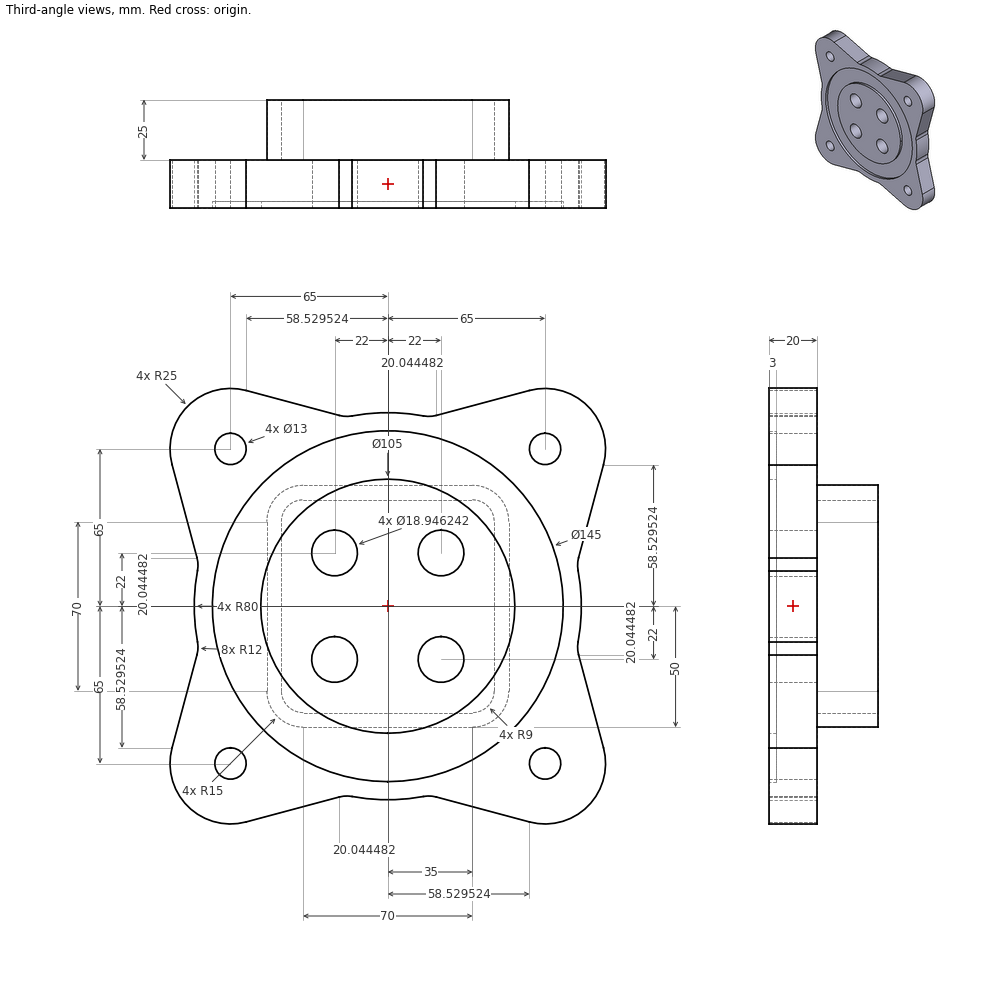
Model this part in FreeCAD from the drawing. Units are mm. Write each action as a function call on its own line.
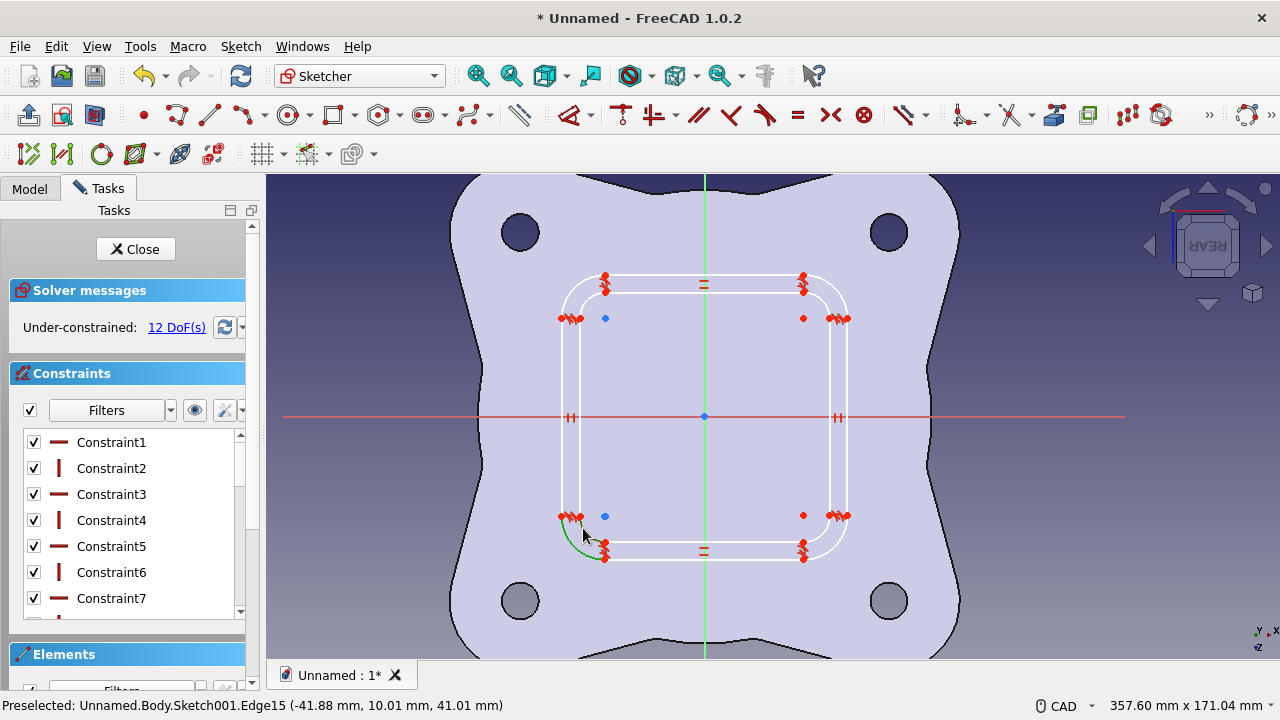
click(621, 116)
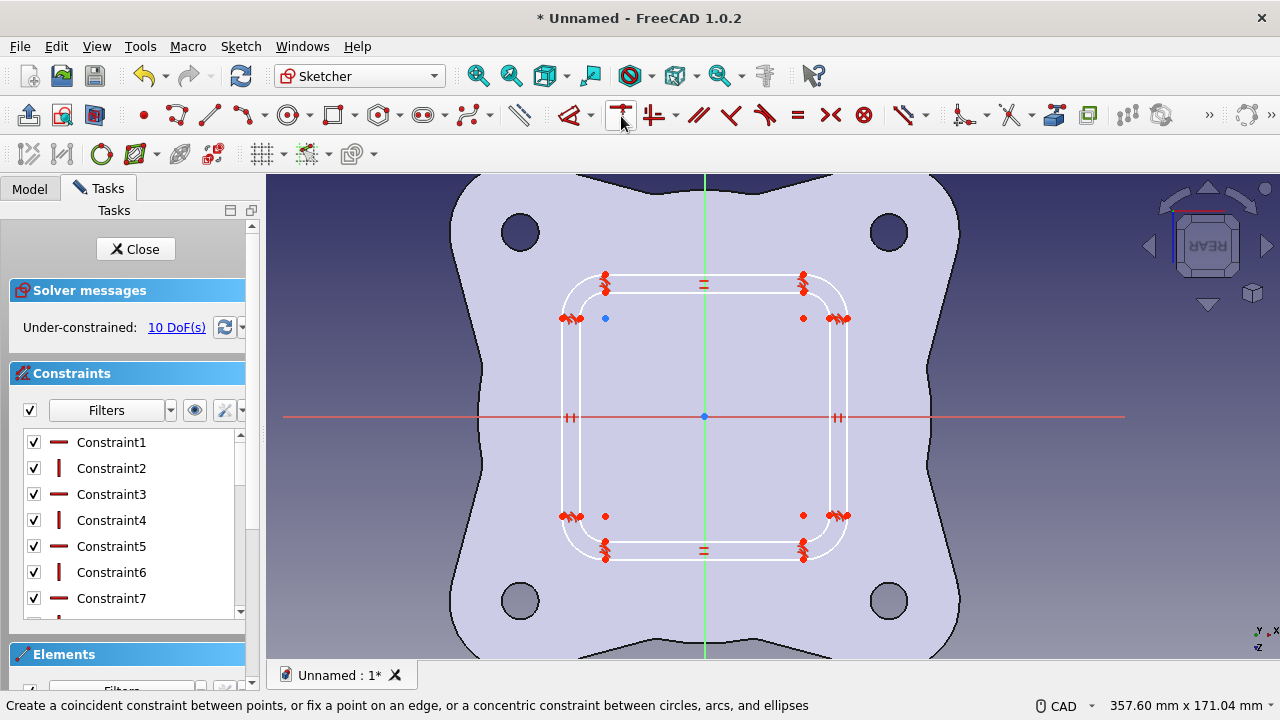
click(586, 280)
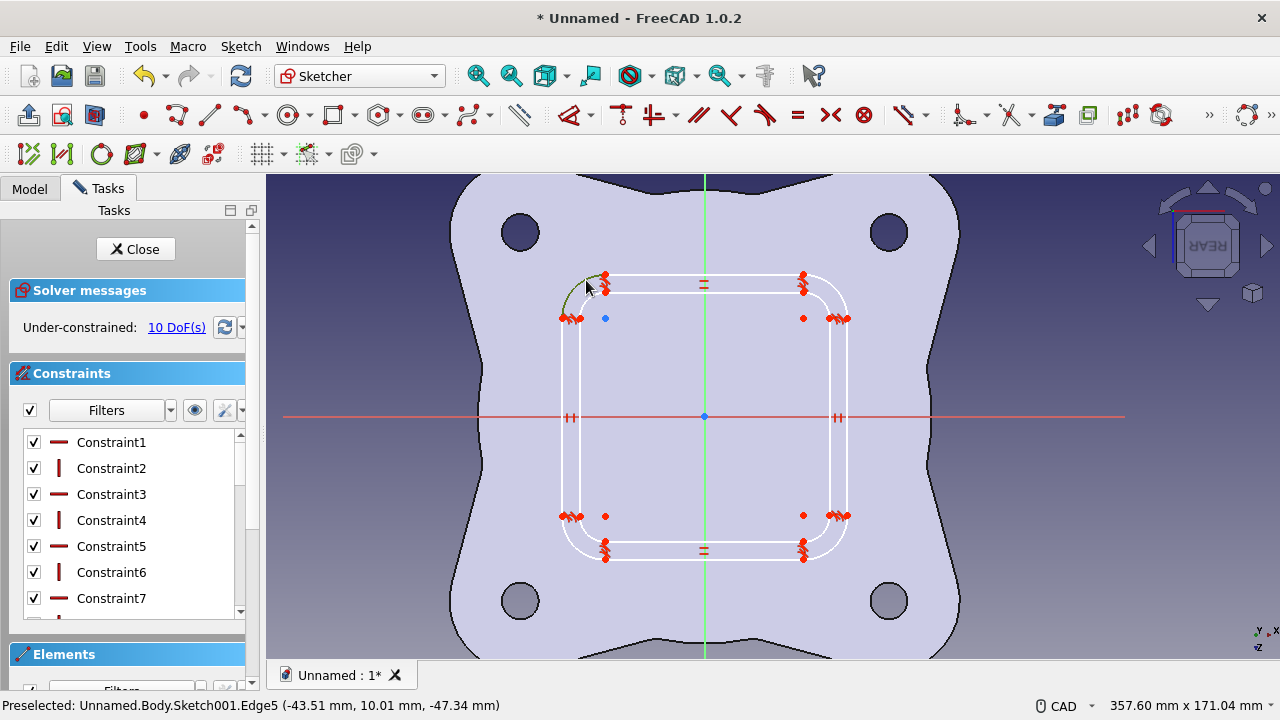
click(567, 536)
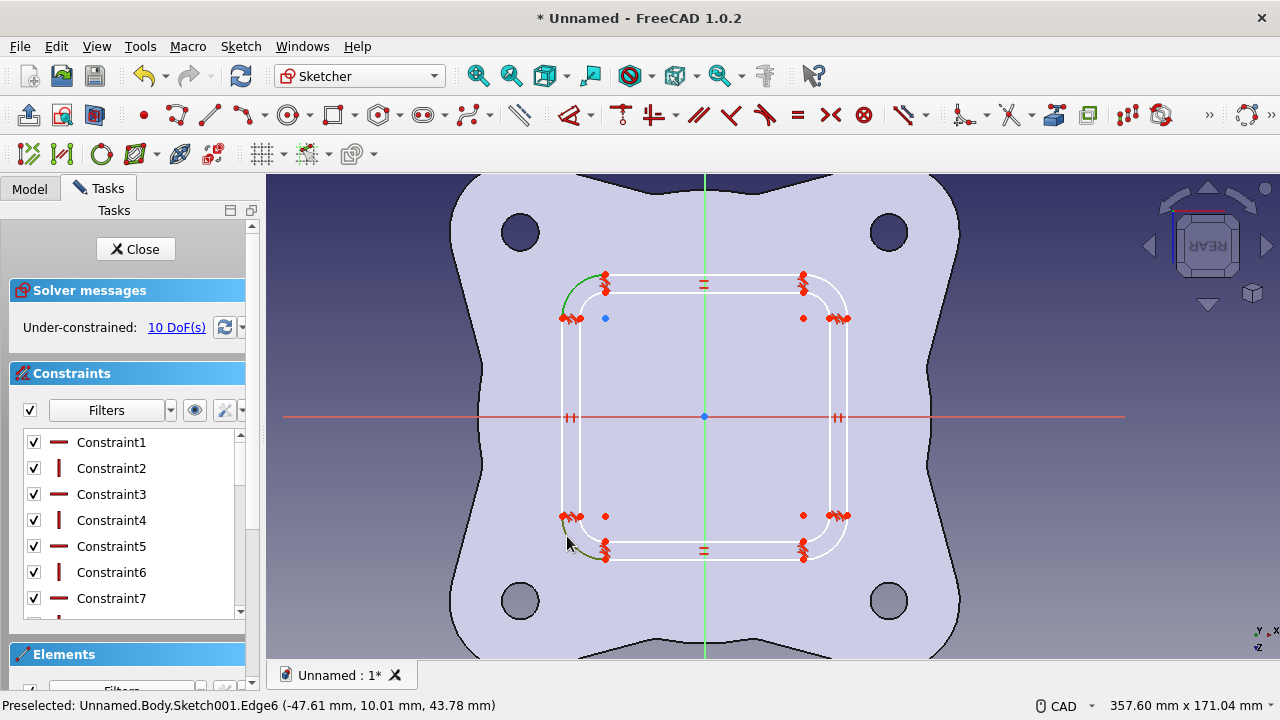
click(824, 555)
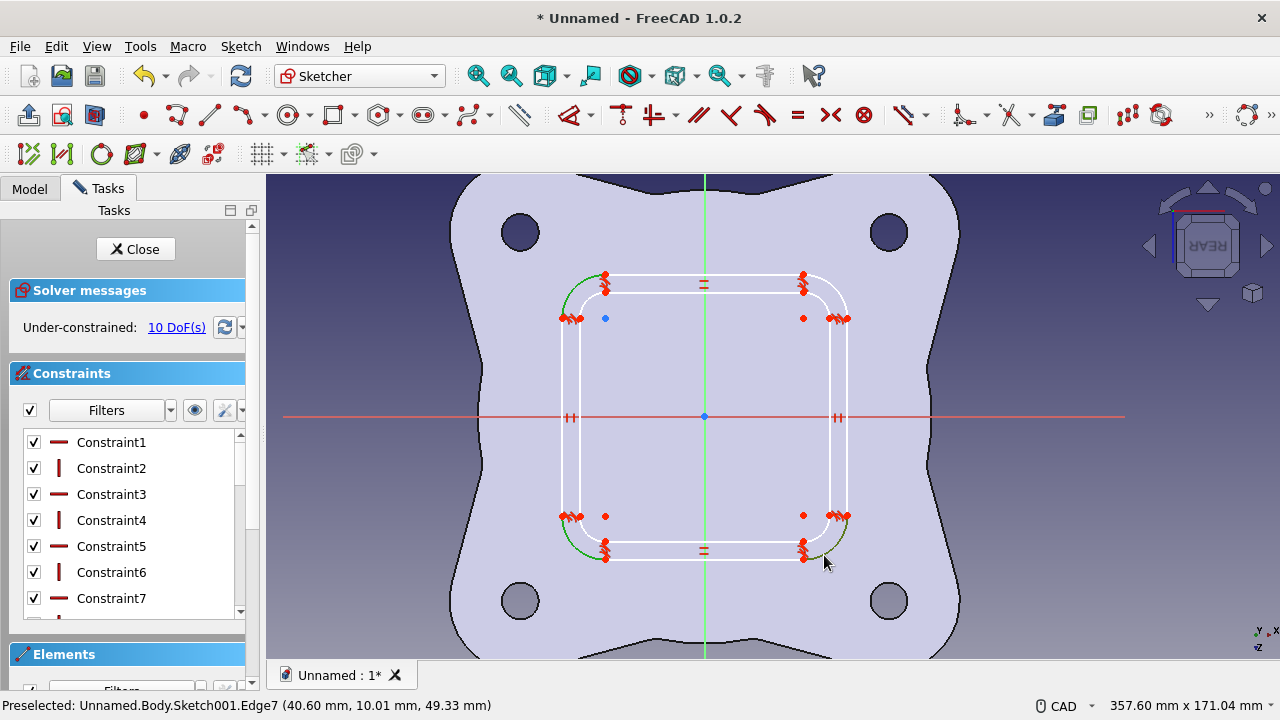
click(843, 299)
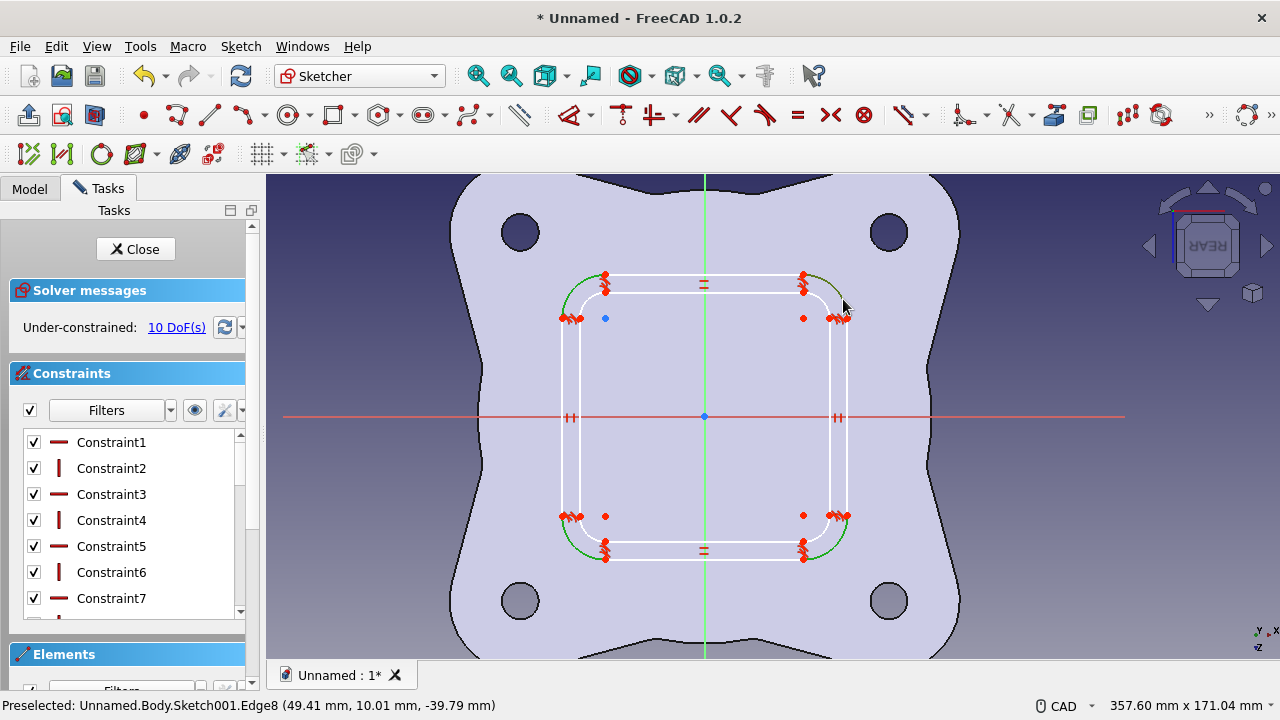
click(798, 116)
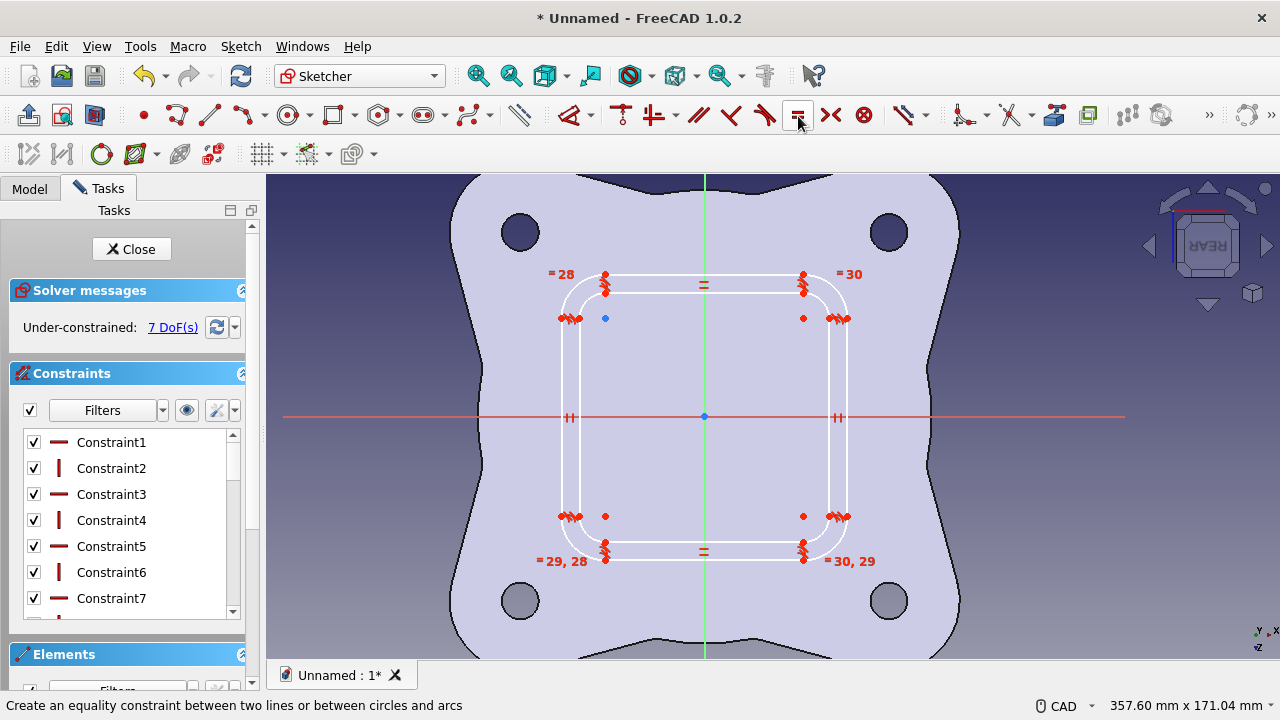
click(826, 307)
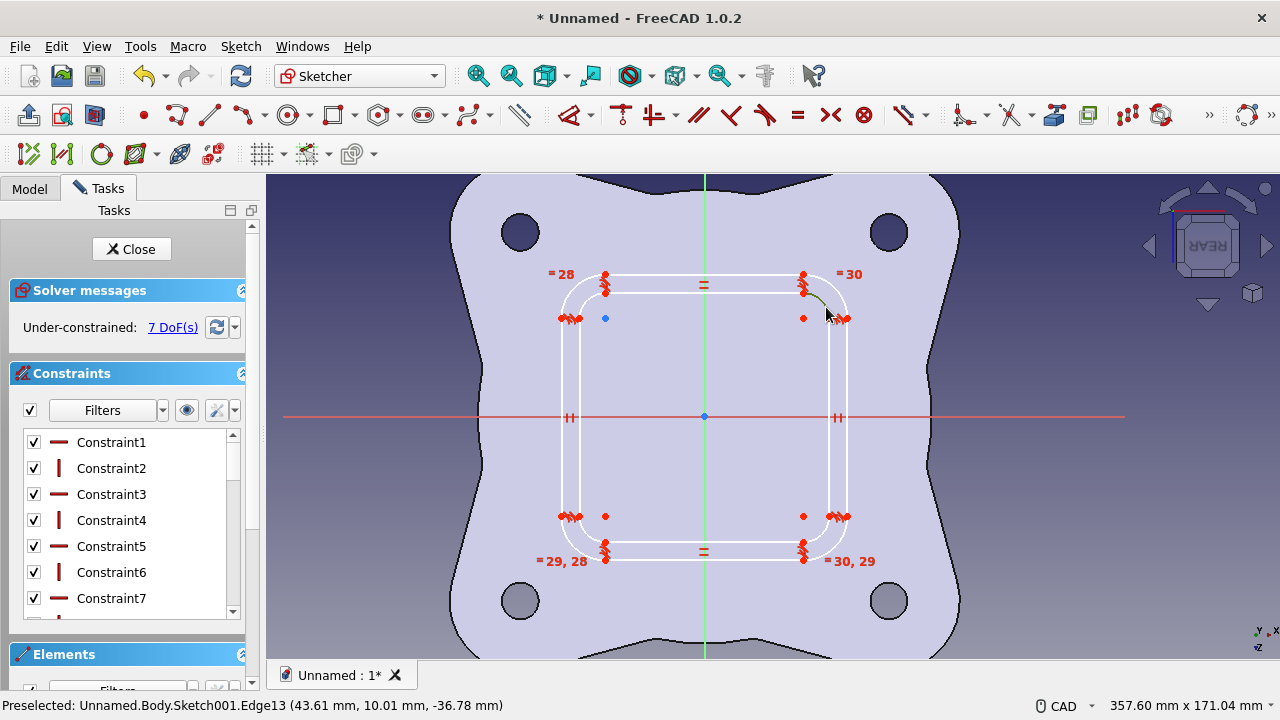
click(594, 296)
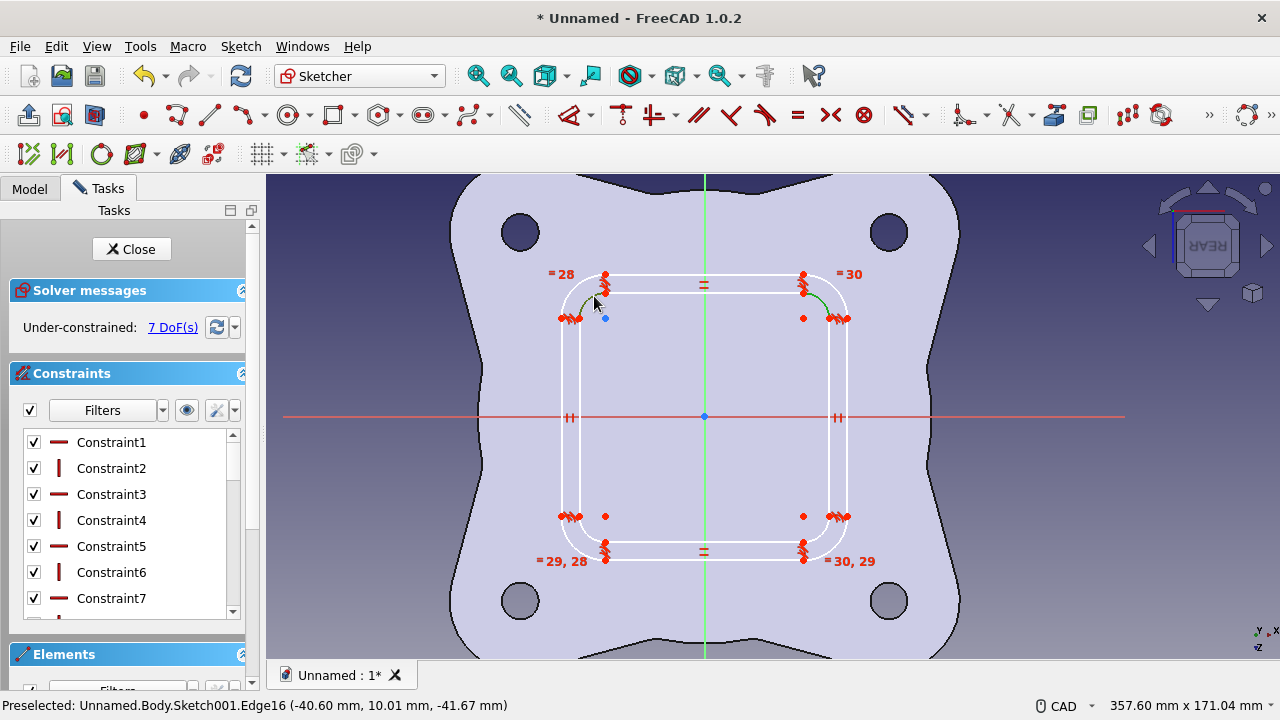
click(798, 116)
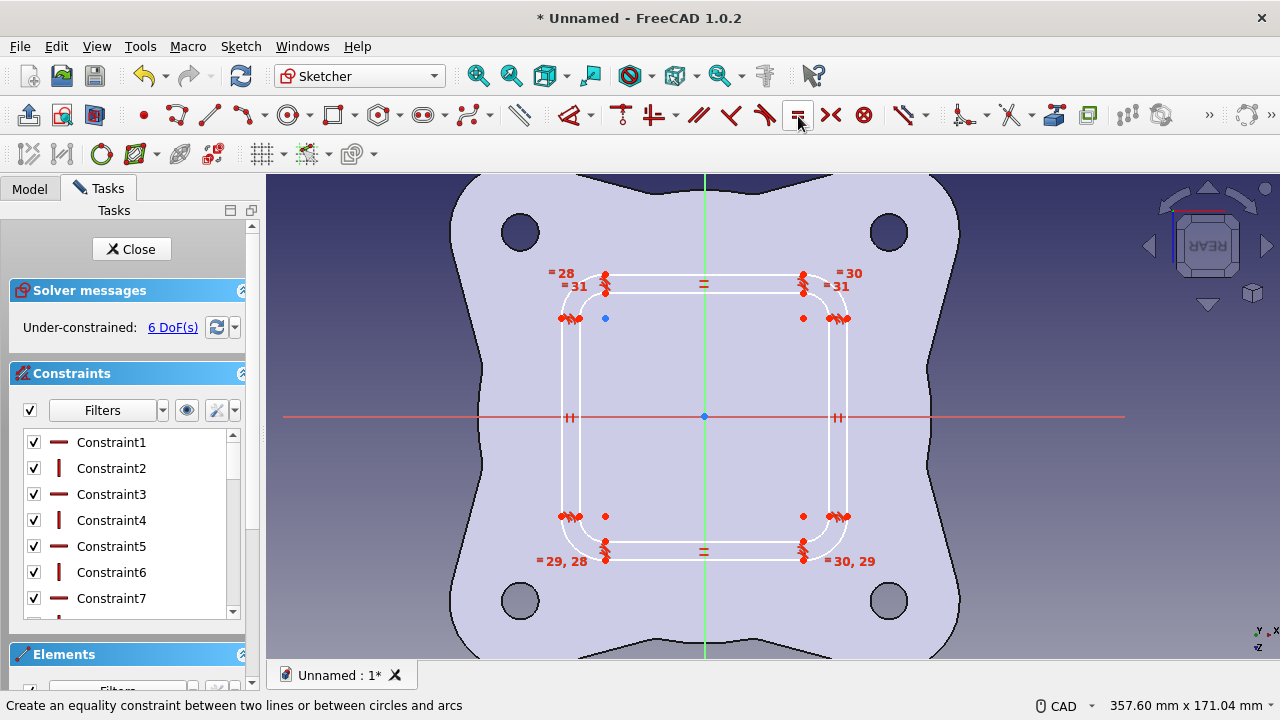
click(568, 116)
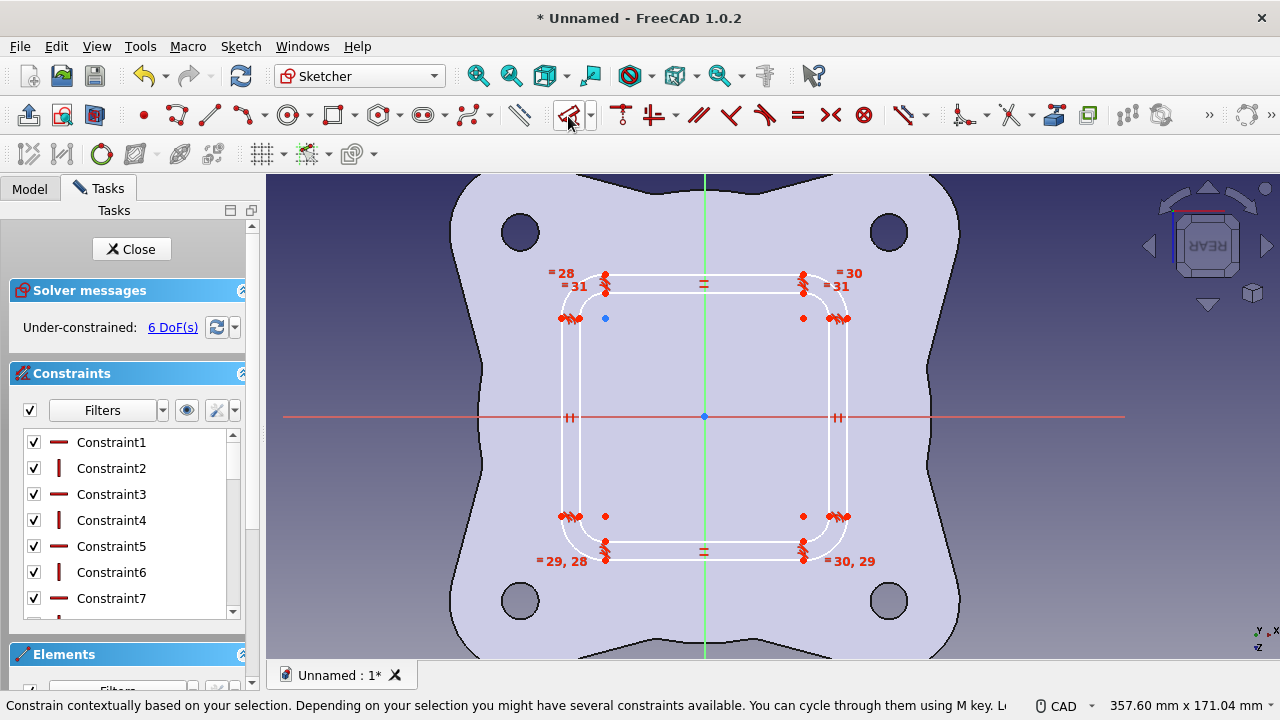
click(585, 280)
click(570, 252)